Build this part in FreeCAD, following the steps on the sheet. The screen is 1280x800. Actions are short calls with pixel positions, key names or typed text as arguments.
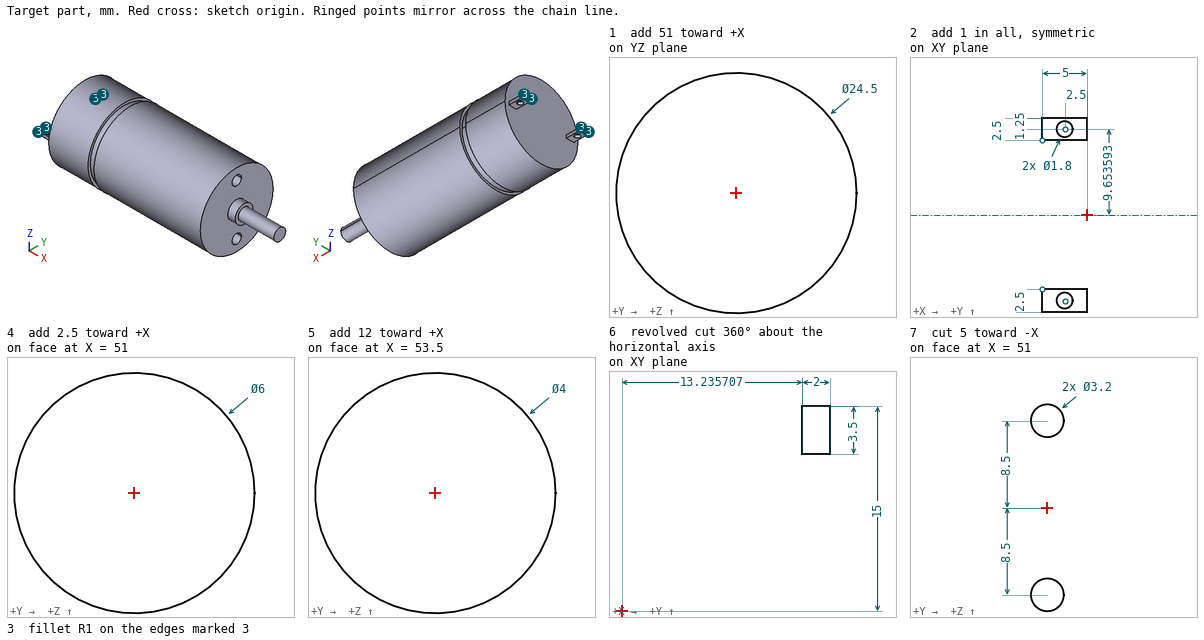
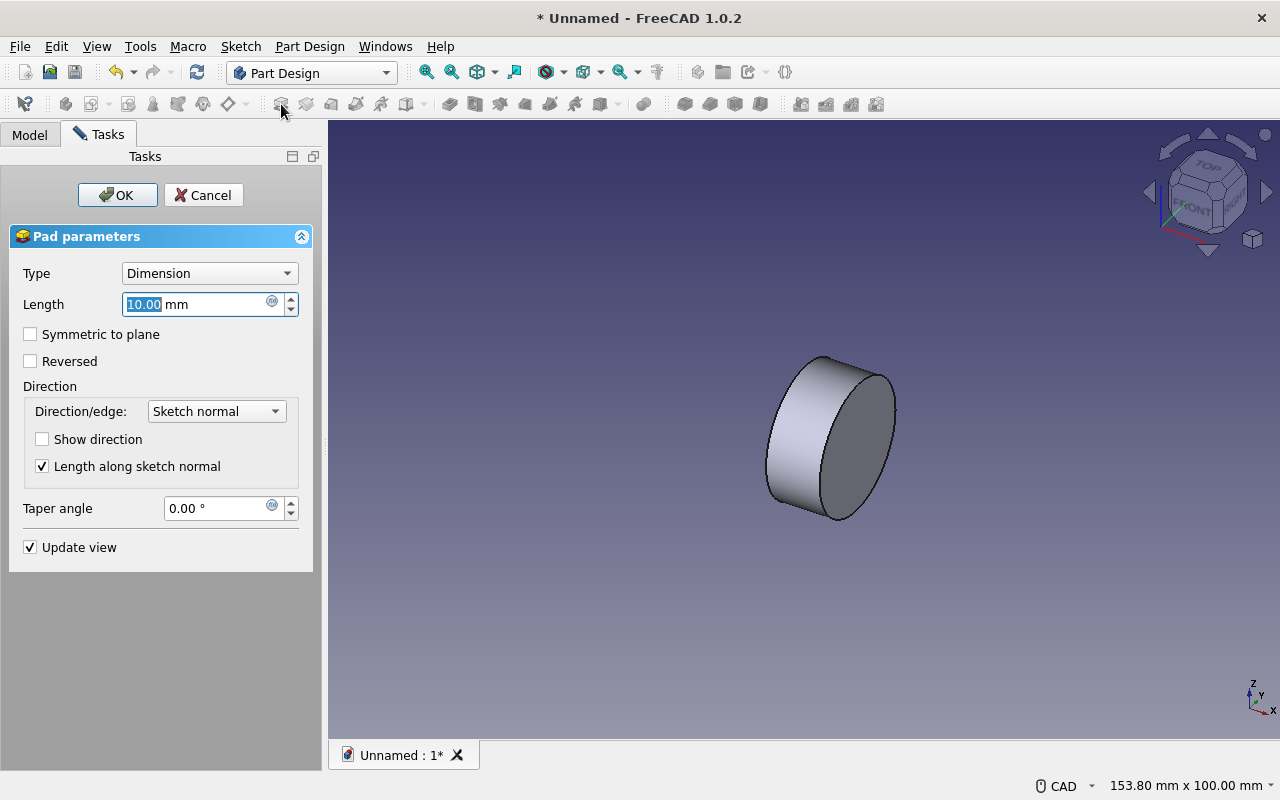
text(51)
key(Tab)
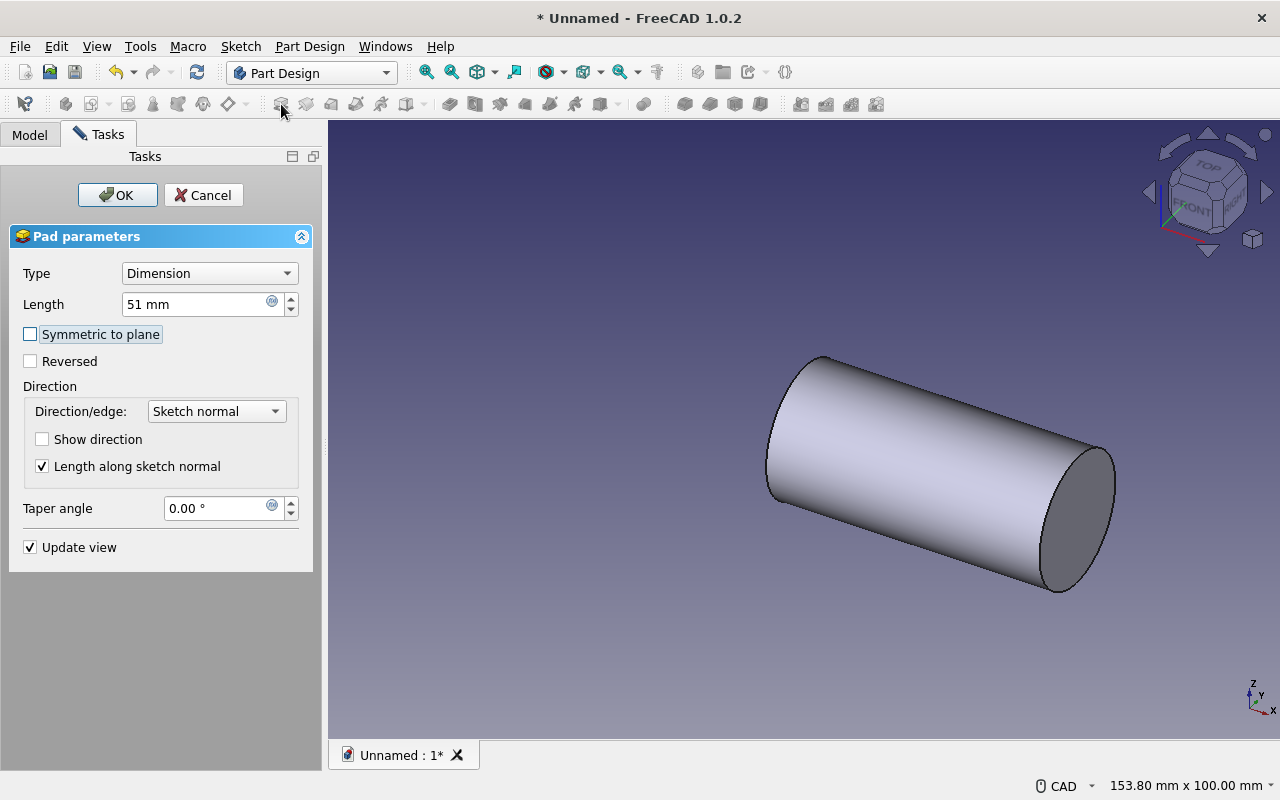
click(118, 195)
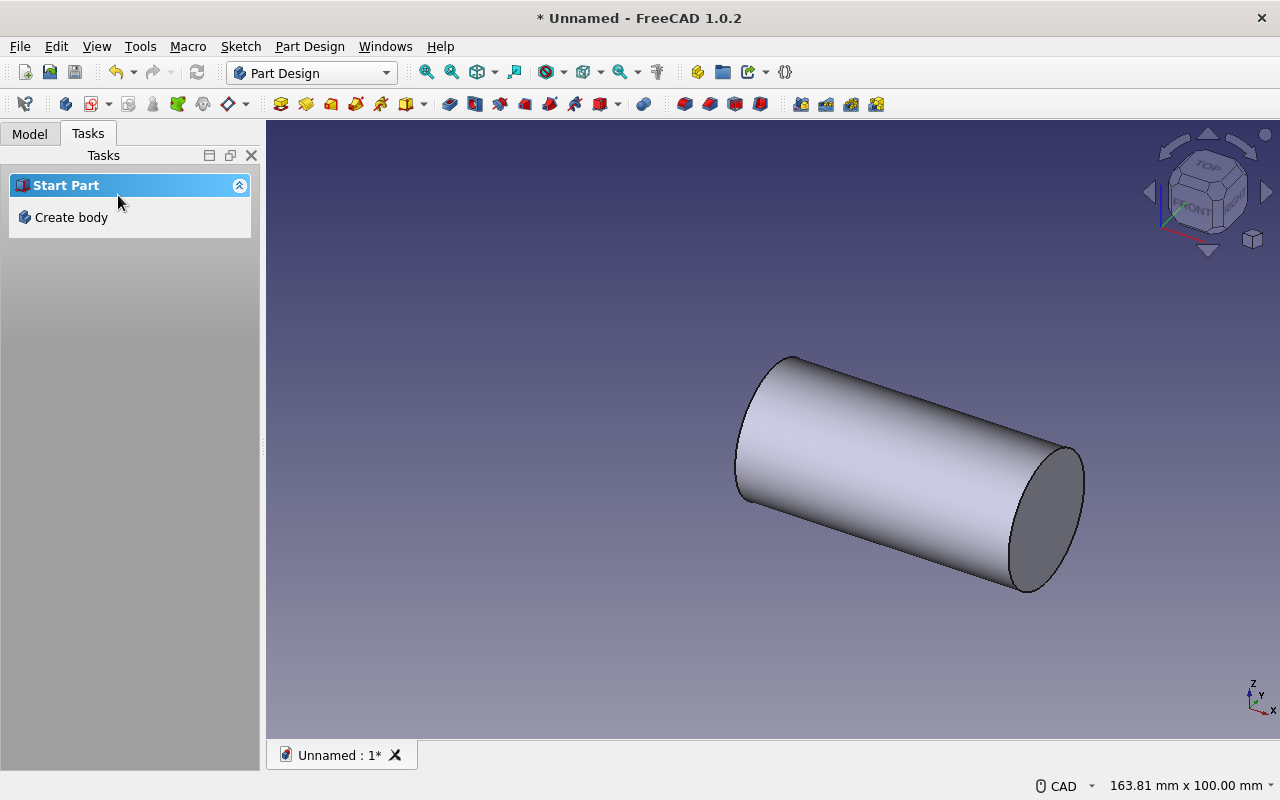
click(90, 104)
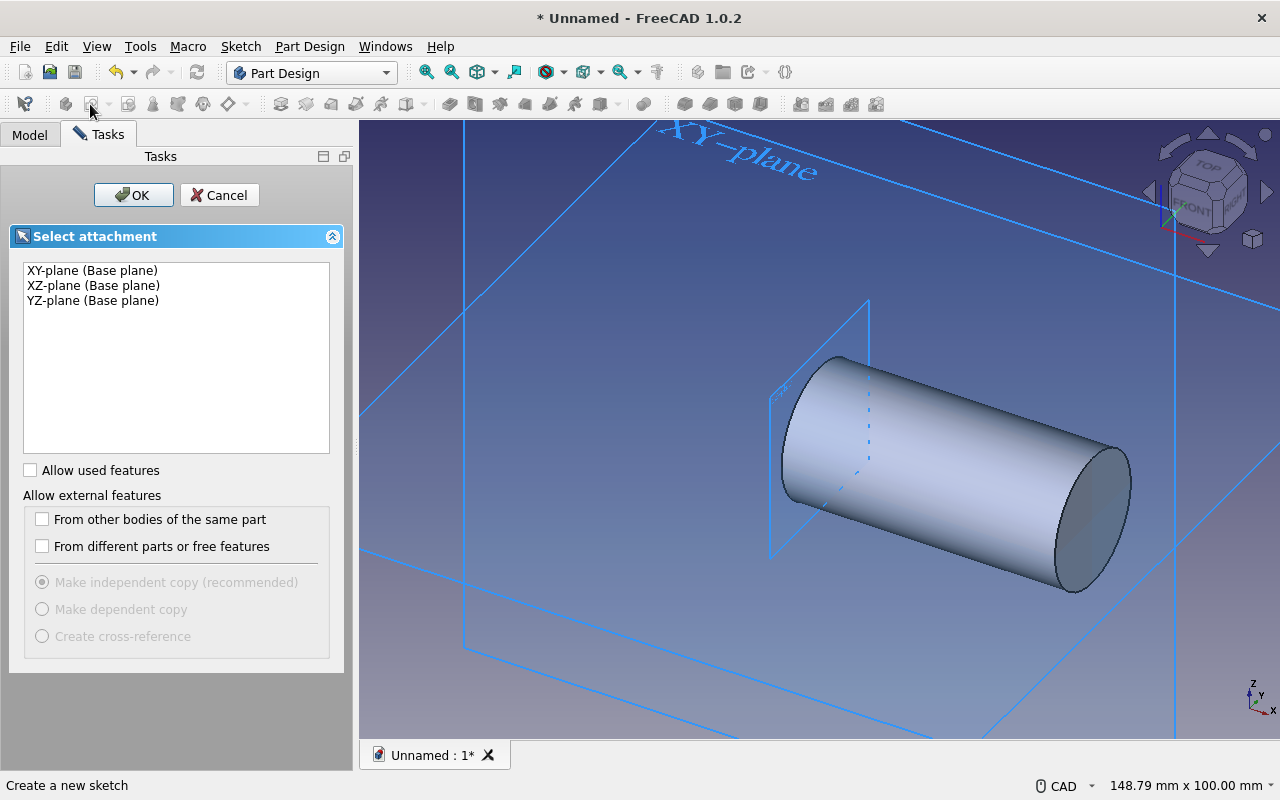
click(84, 270)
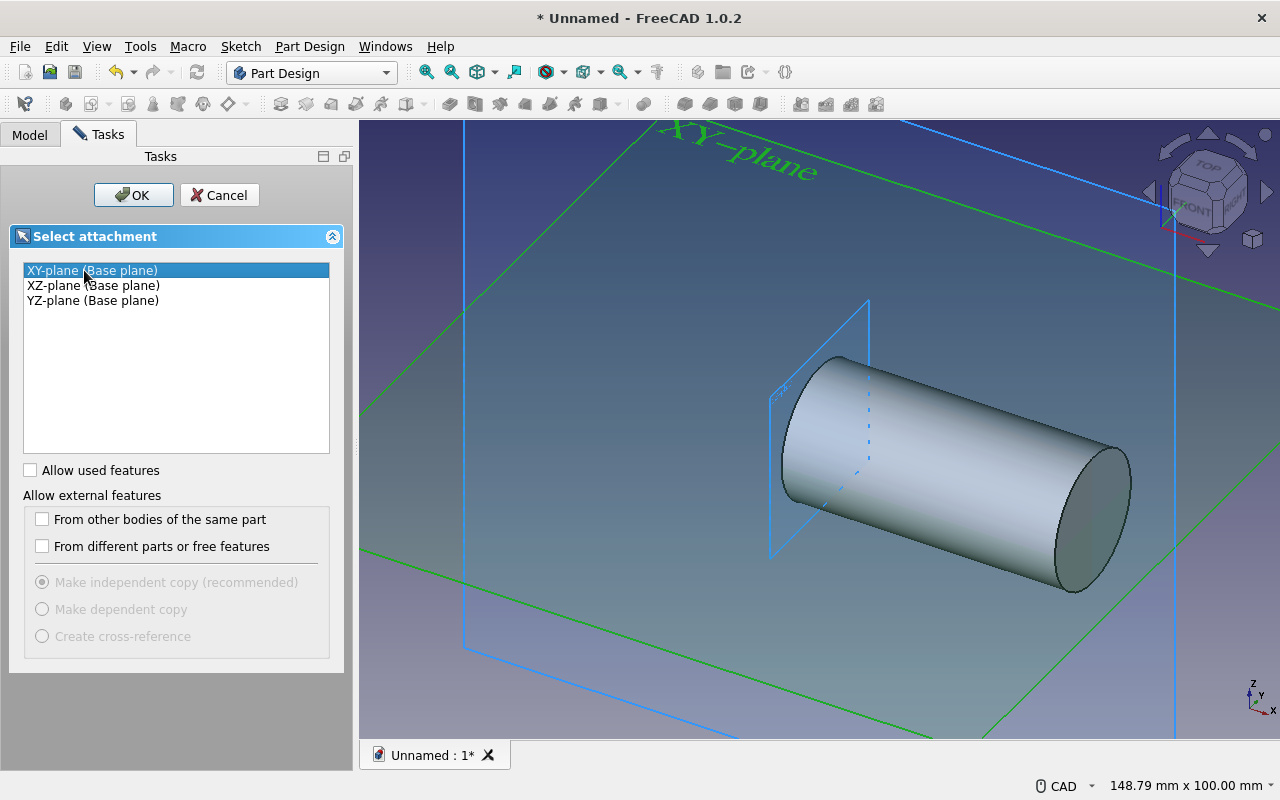
click(134, 195)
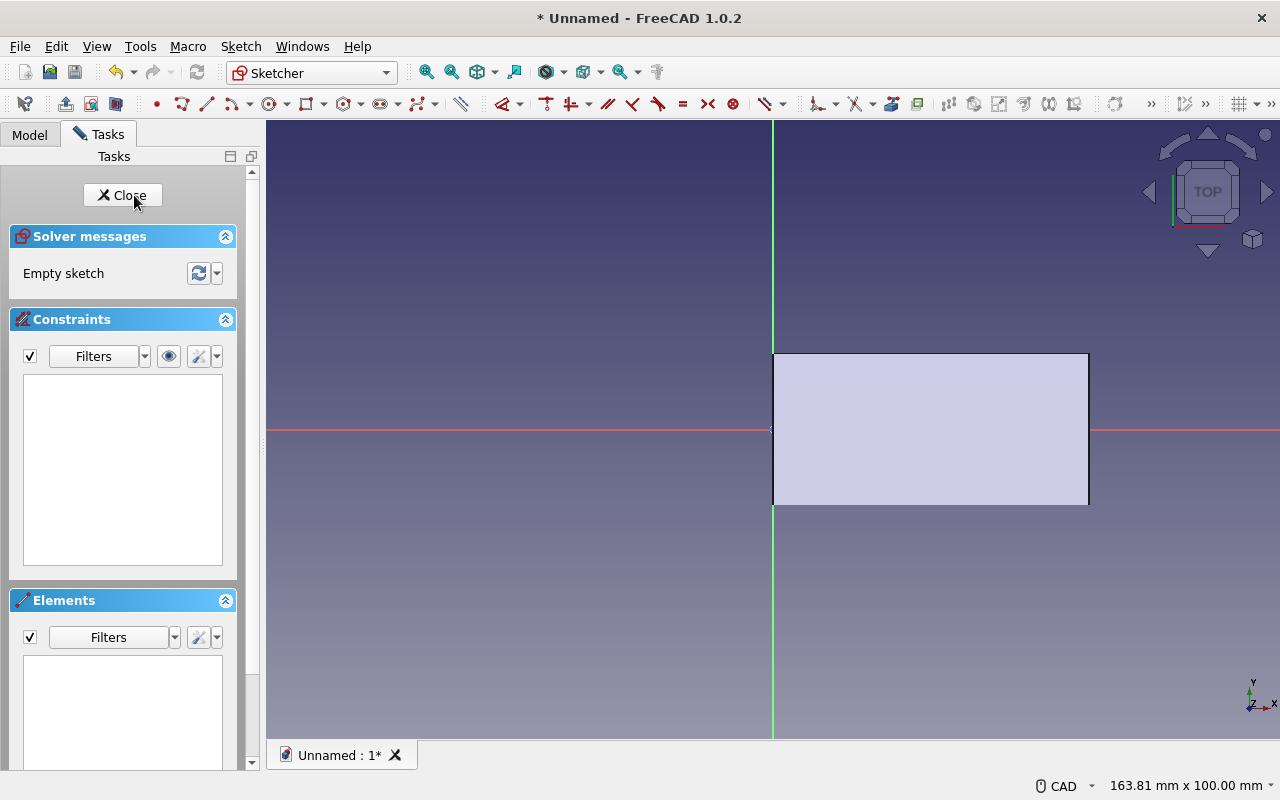
click(116, 104)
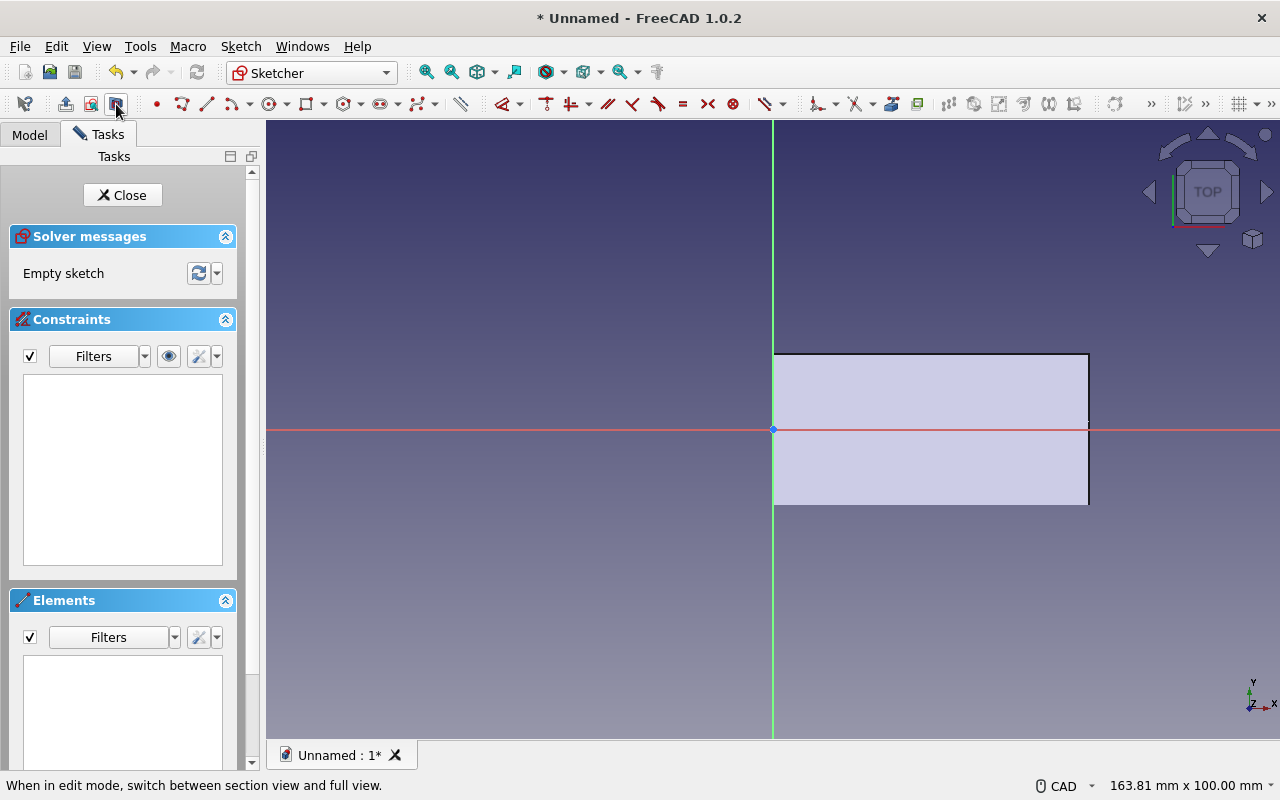
scroll(788, 429, up, 5)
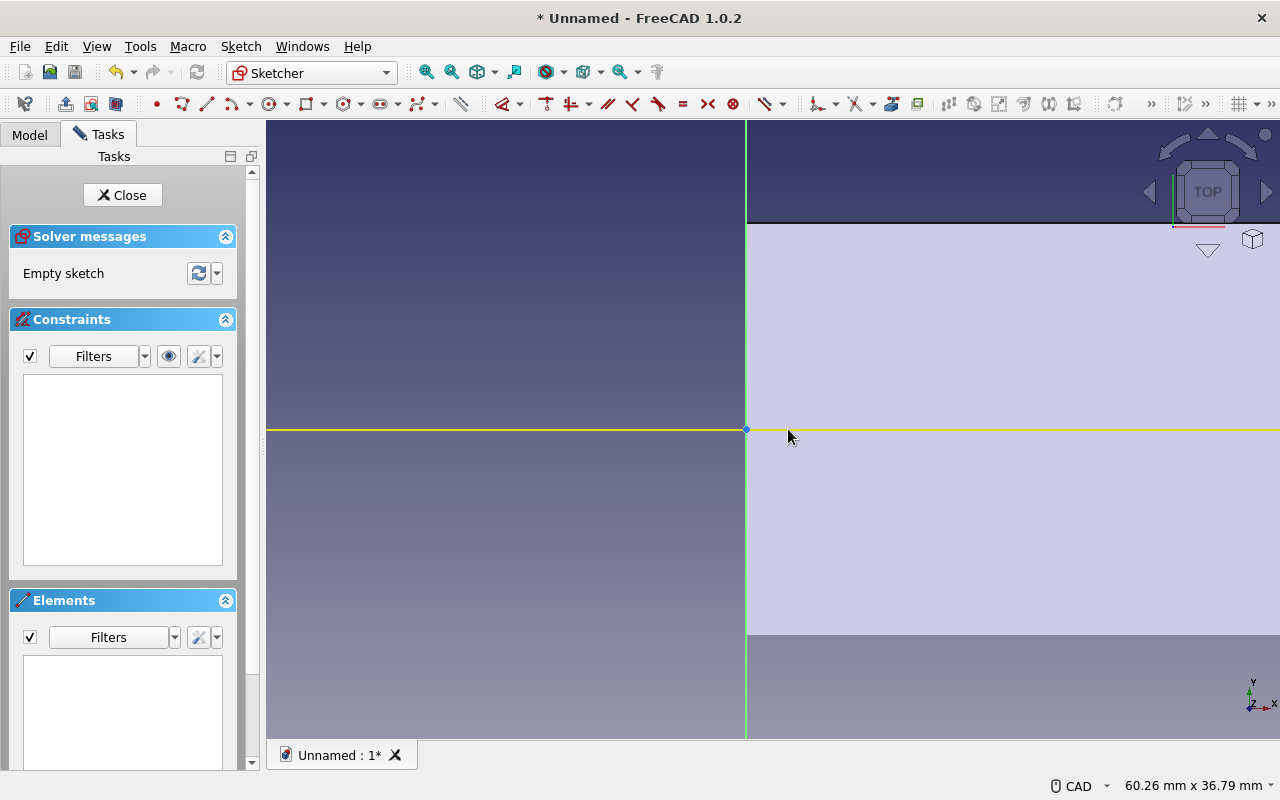
click(306, 104)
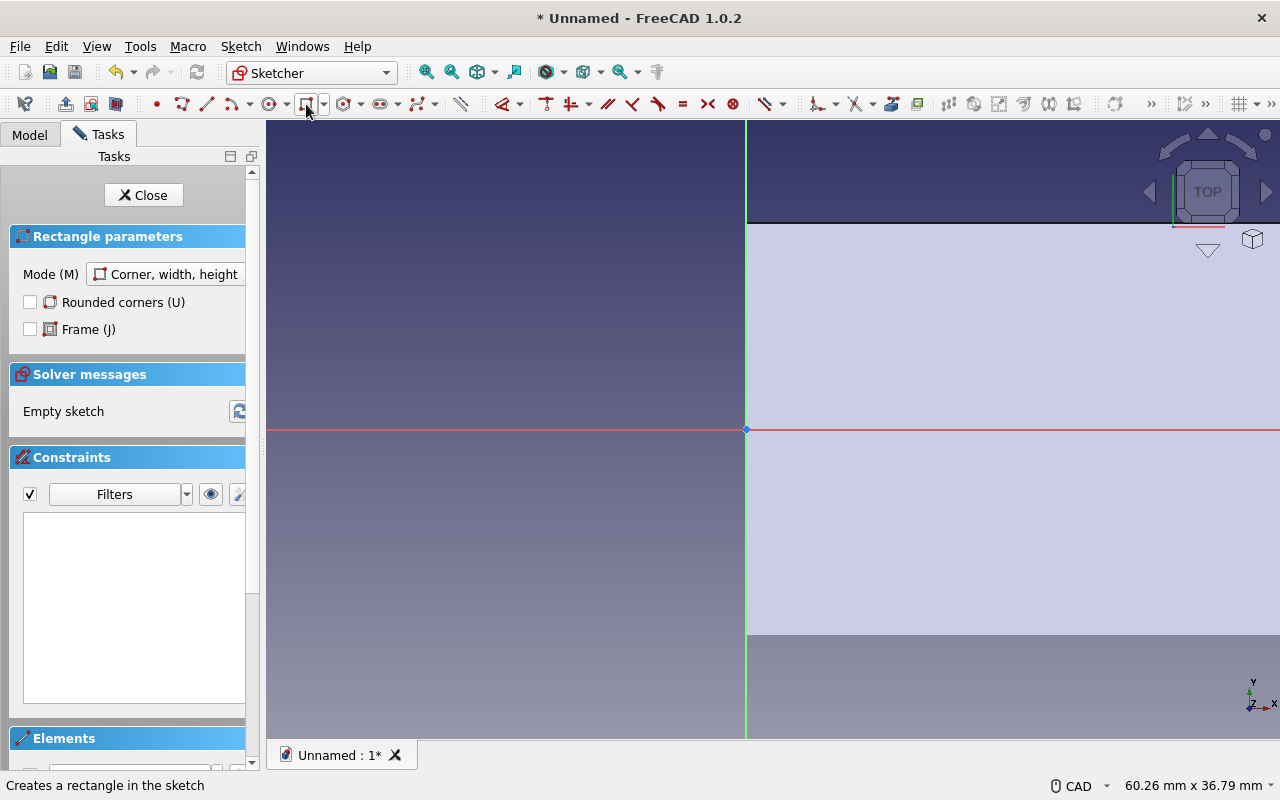
click(662, 246)
click(746, 288)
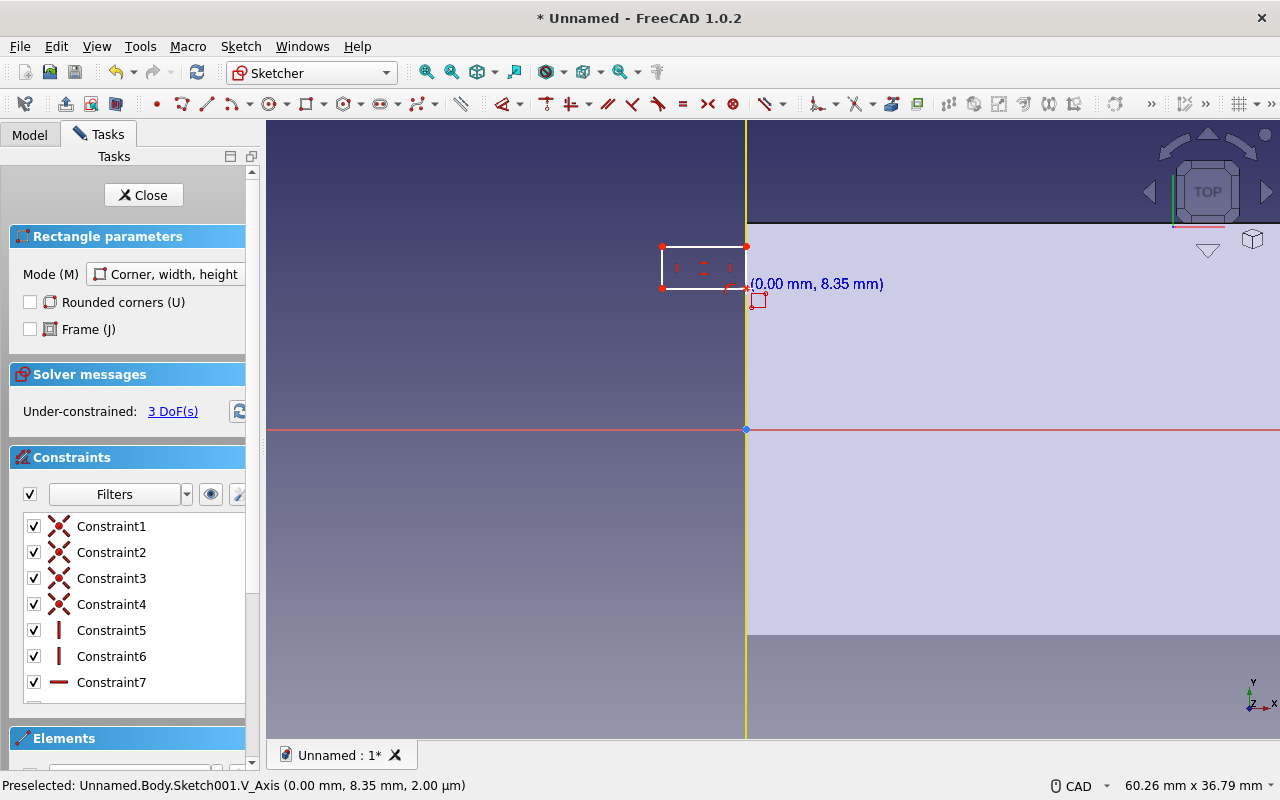
click(662, 571)
click(746, 613)